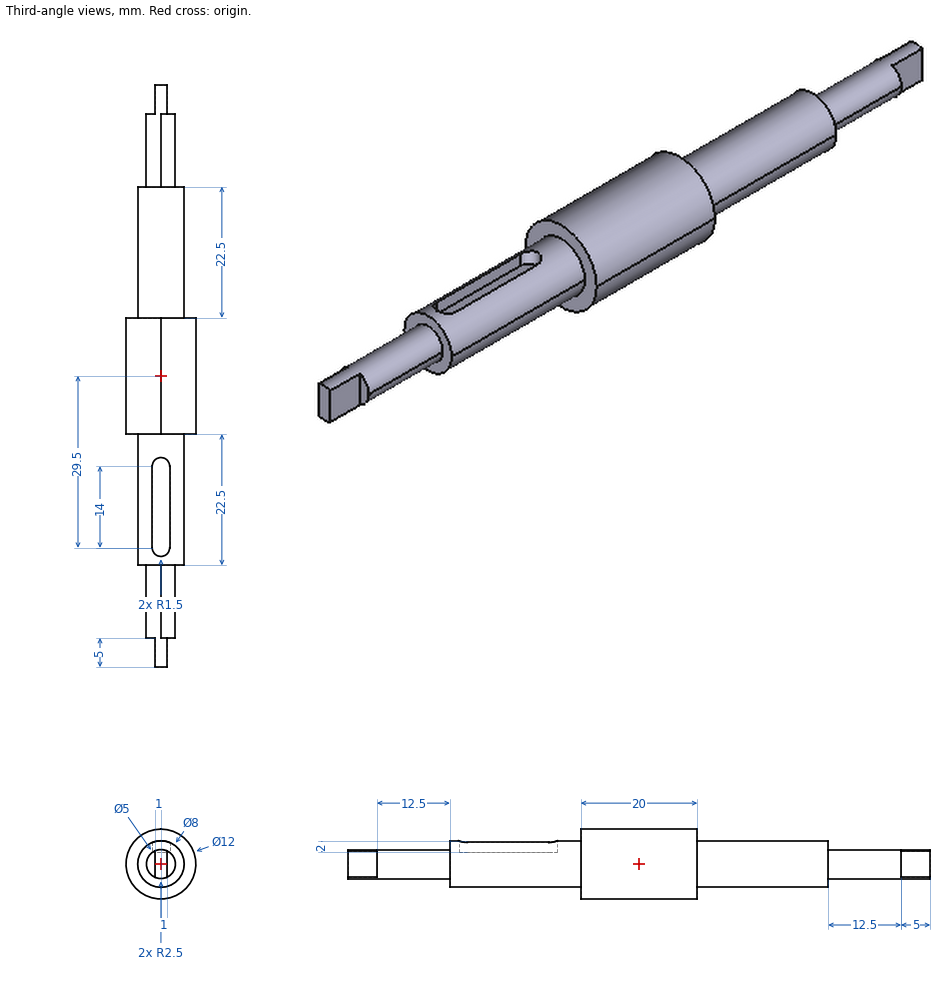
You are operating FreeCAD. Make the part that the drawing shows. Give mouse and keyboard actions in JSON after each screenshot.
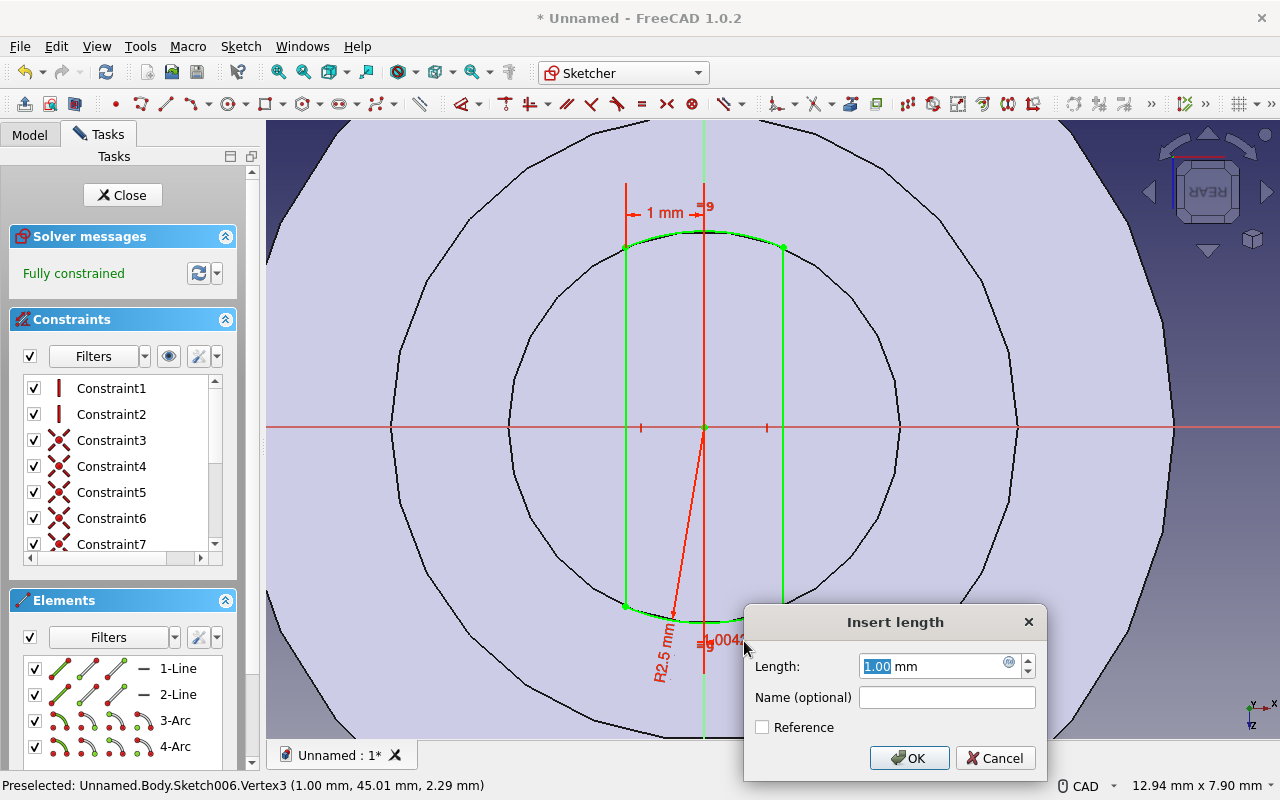
{"action": "type", "text": "1"}
{"action": "key", "text": "Return"}
{"action": "key", "text": "Escape"}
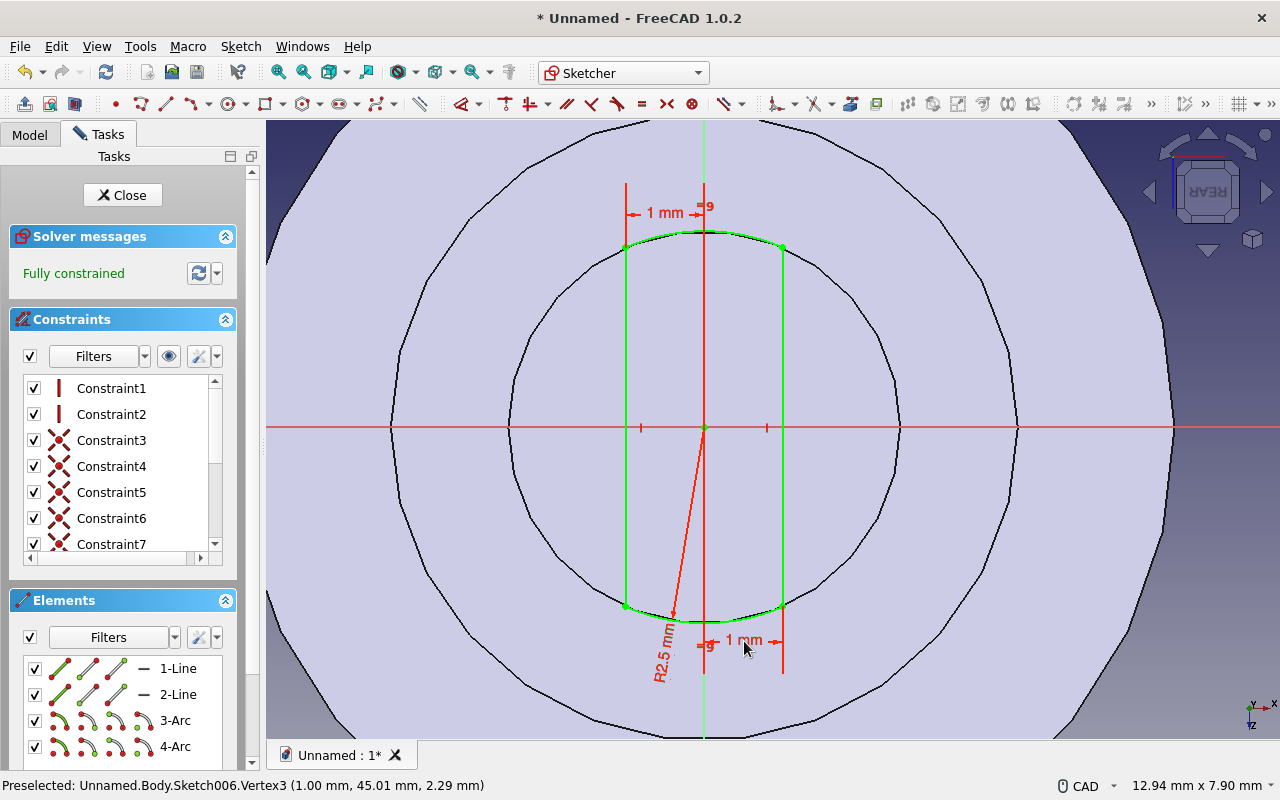
{"action": "left_click", "coordinate": [123, 195]}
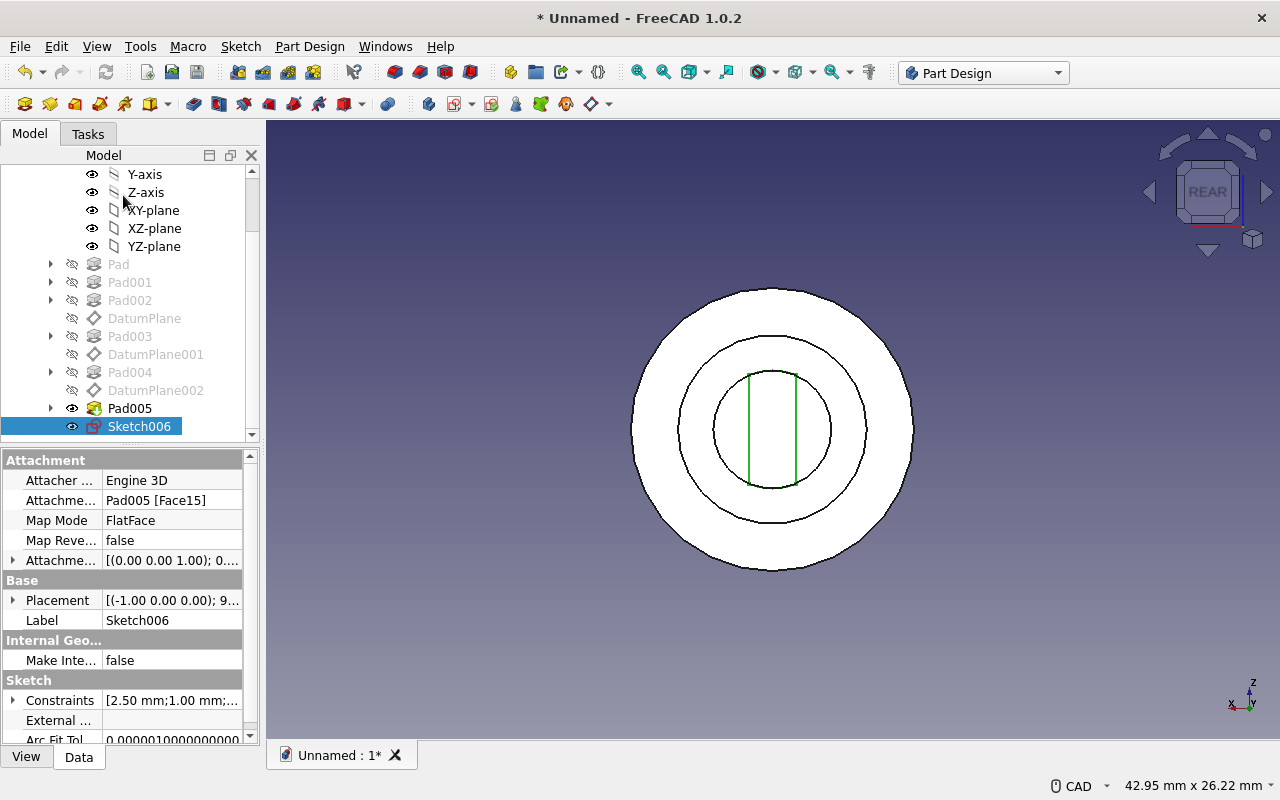
{"action": "left_click", "coordinate": [25, 104]}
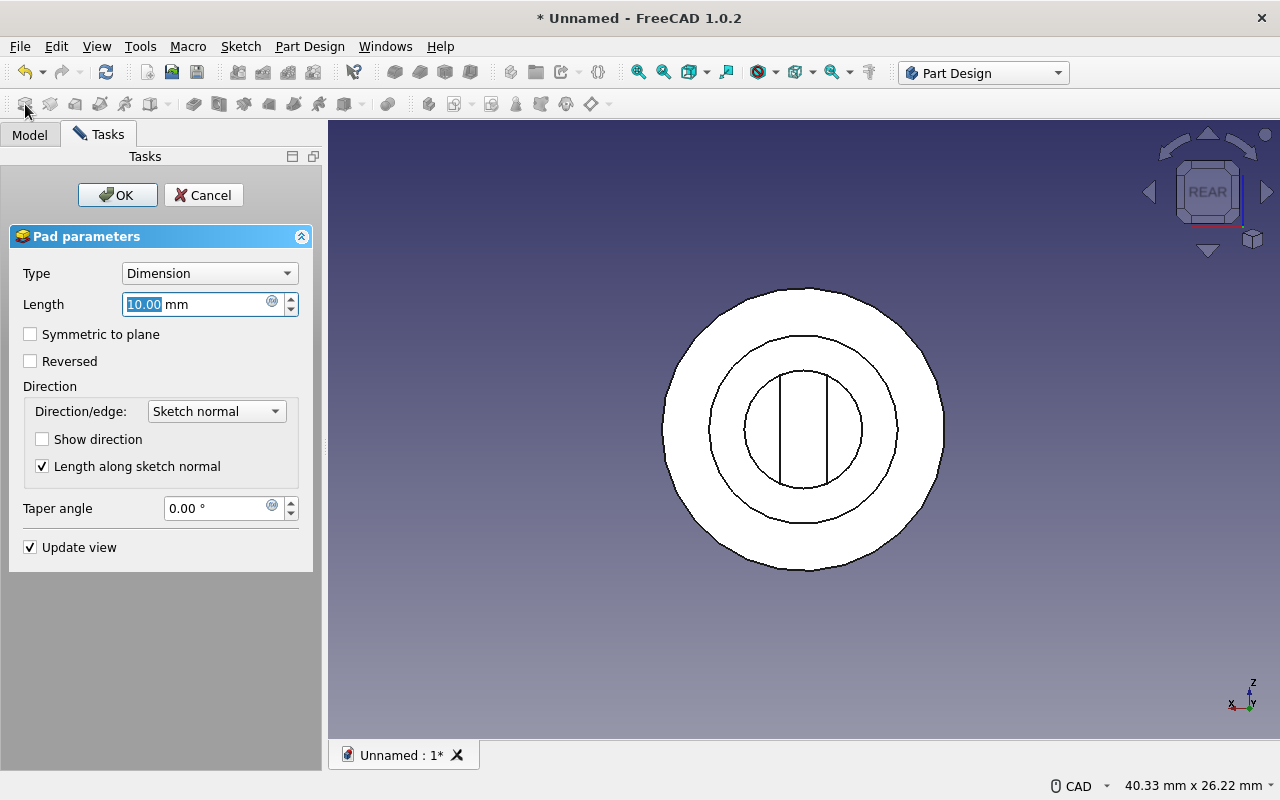
{"action": "type", "text": "5"}
{"action": "key", "text": "Tab"}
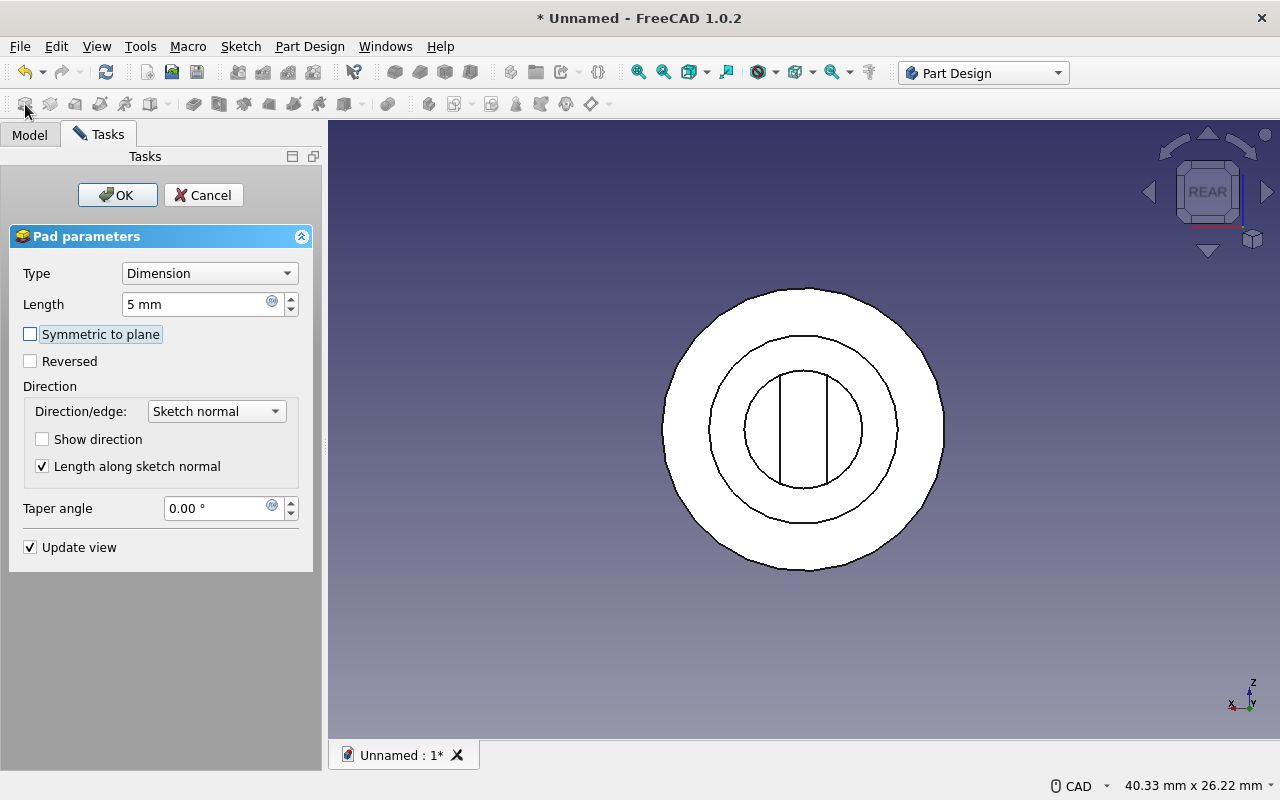
{"action": "left_click", "coordinate": [118, 195]}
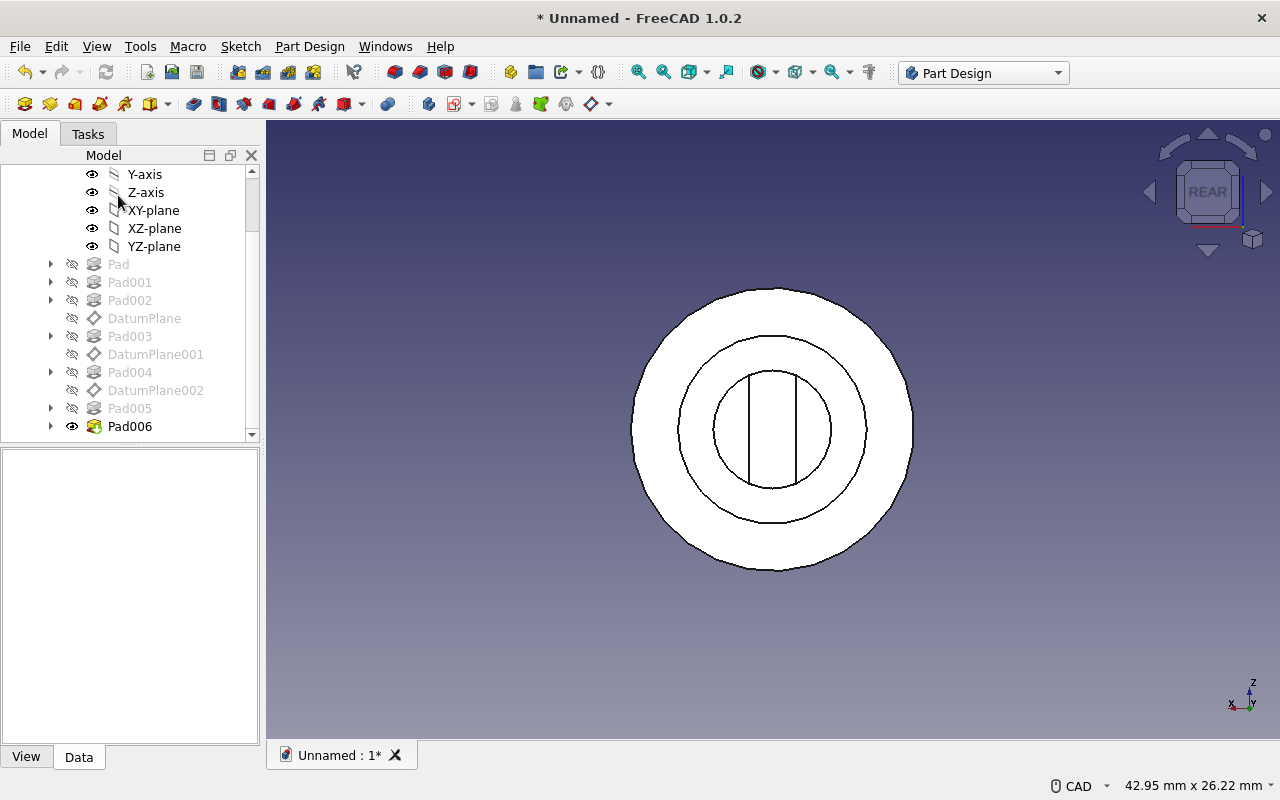
{"action": "scroll", "coordinate": [161, 296], "scroll_direction": "down", "scroll_amount": 3}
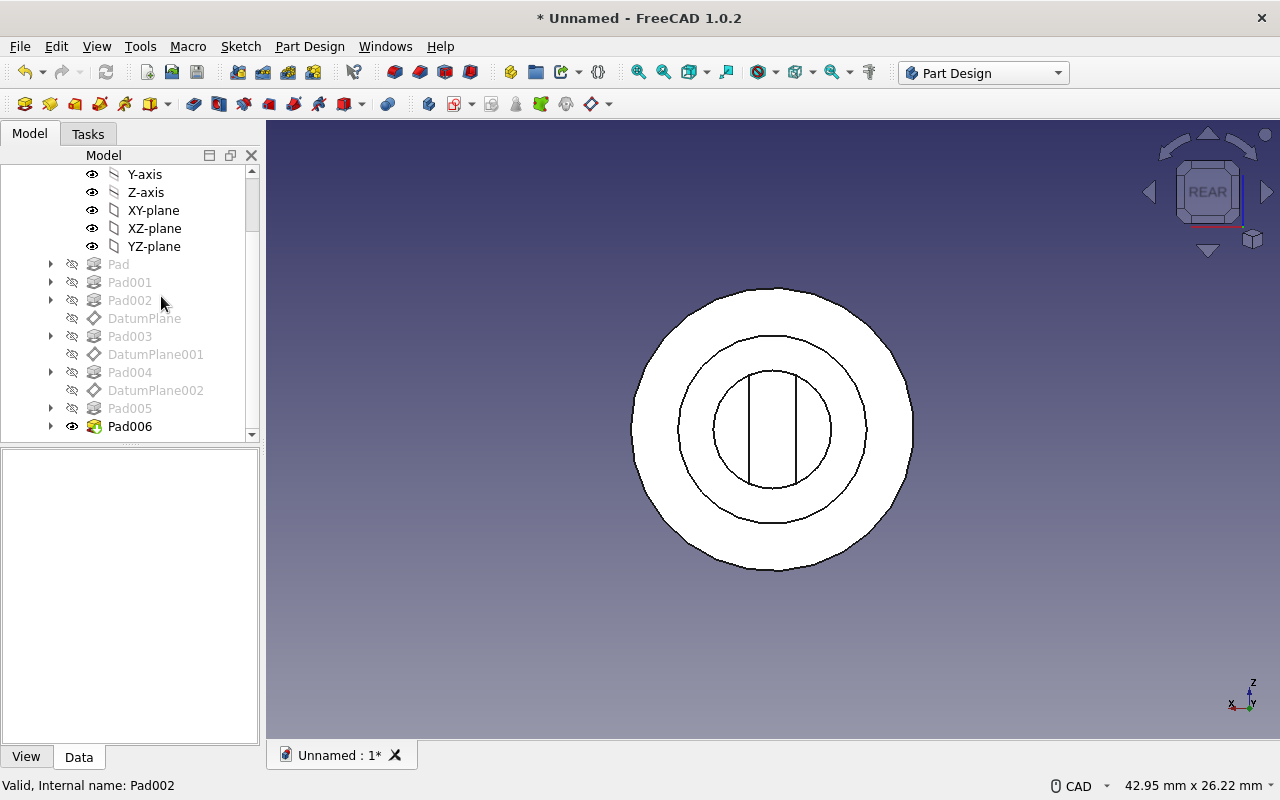
{"action": "scroll", "coordinate": [161, 296], "scroll_direction": "up", "scroll_amount": 15}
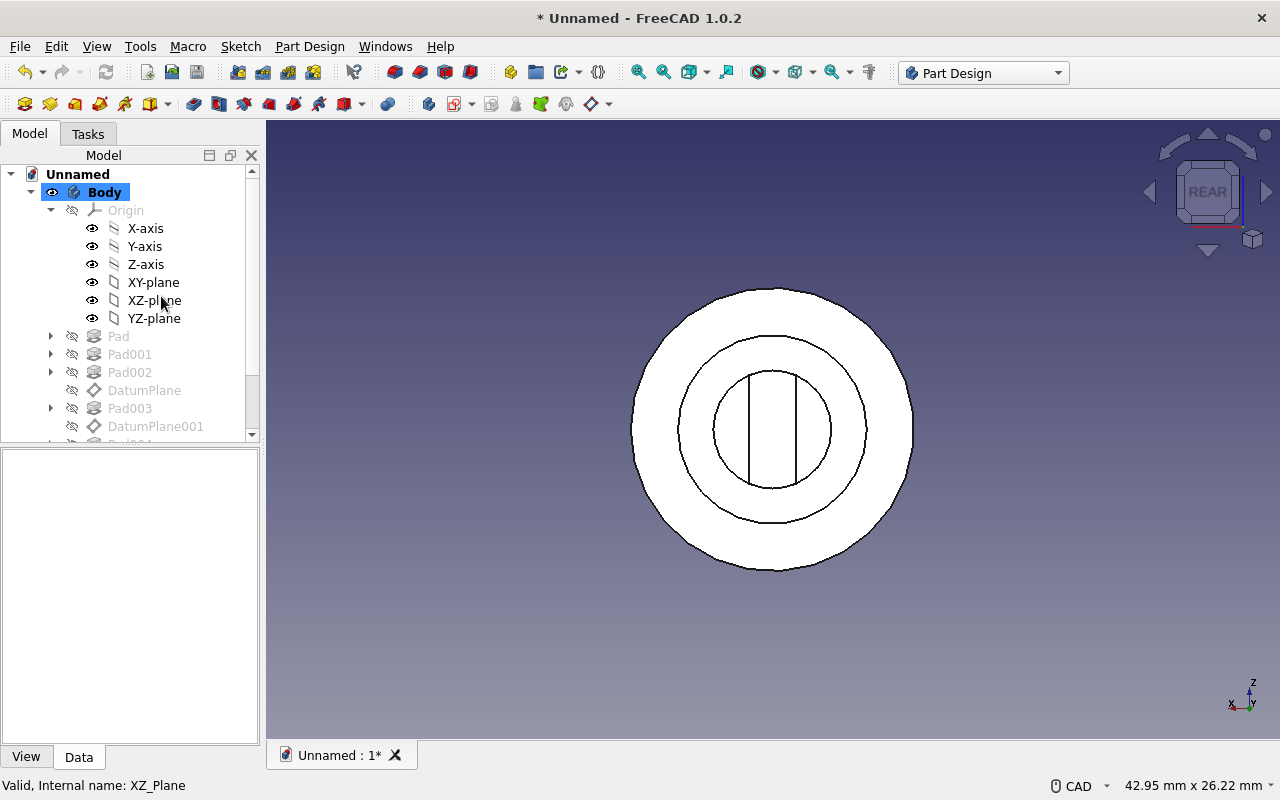
{"action": "left_click", "coordinate": [137, 282]}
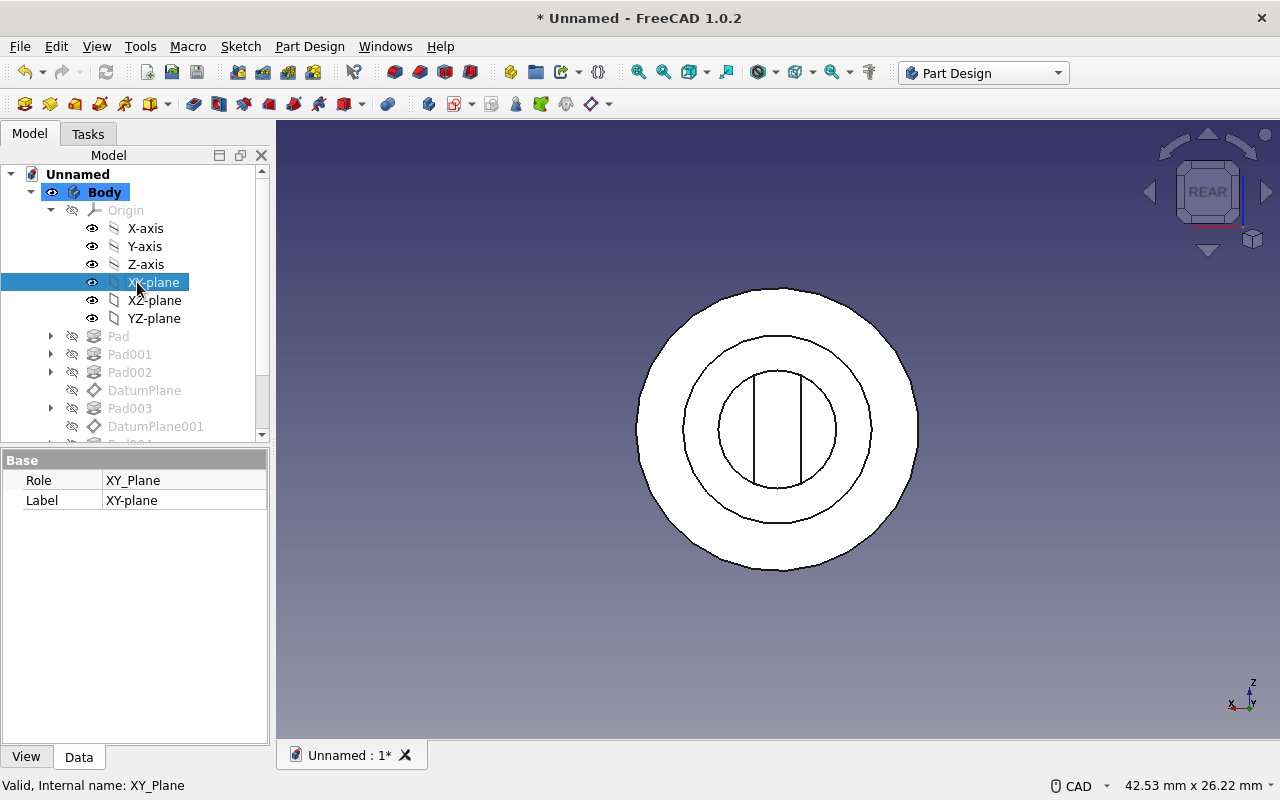
{"action": "left_click", "coordinate": [590, 104]}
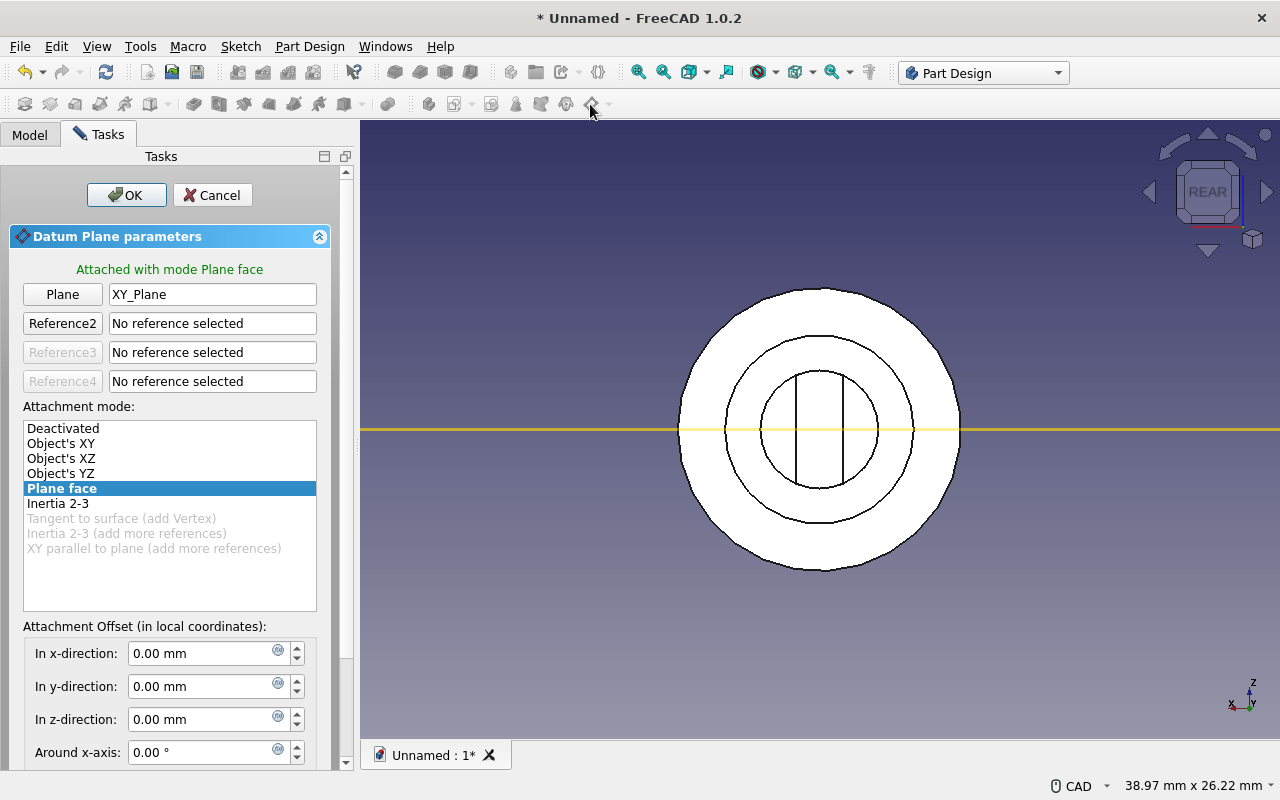
{"action": "triple_click", "coordinate": [210, 720]}